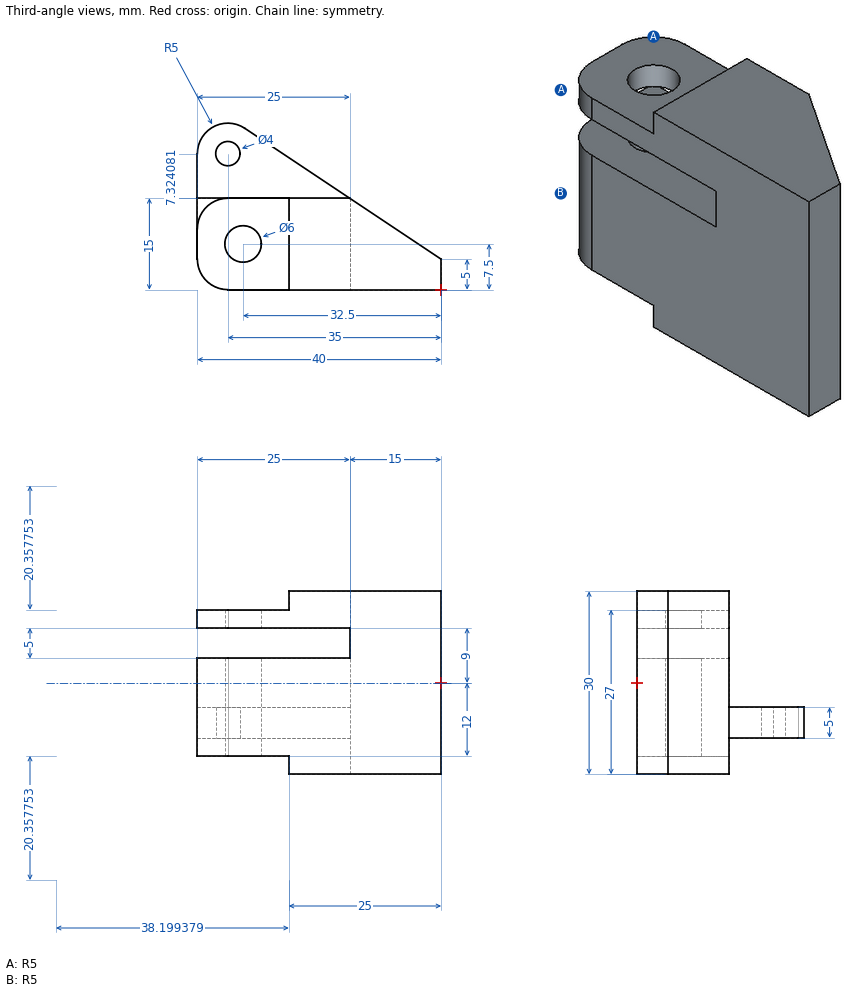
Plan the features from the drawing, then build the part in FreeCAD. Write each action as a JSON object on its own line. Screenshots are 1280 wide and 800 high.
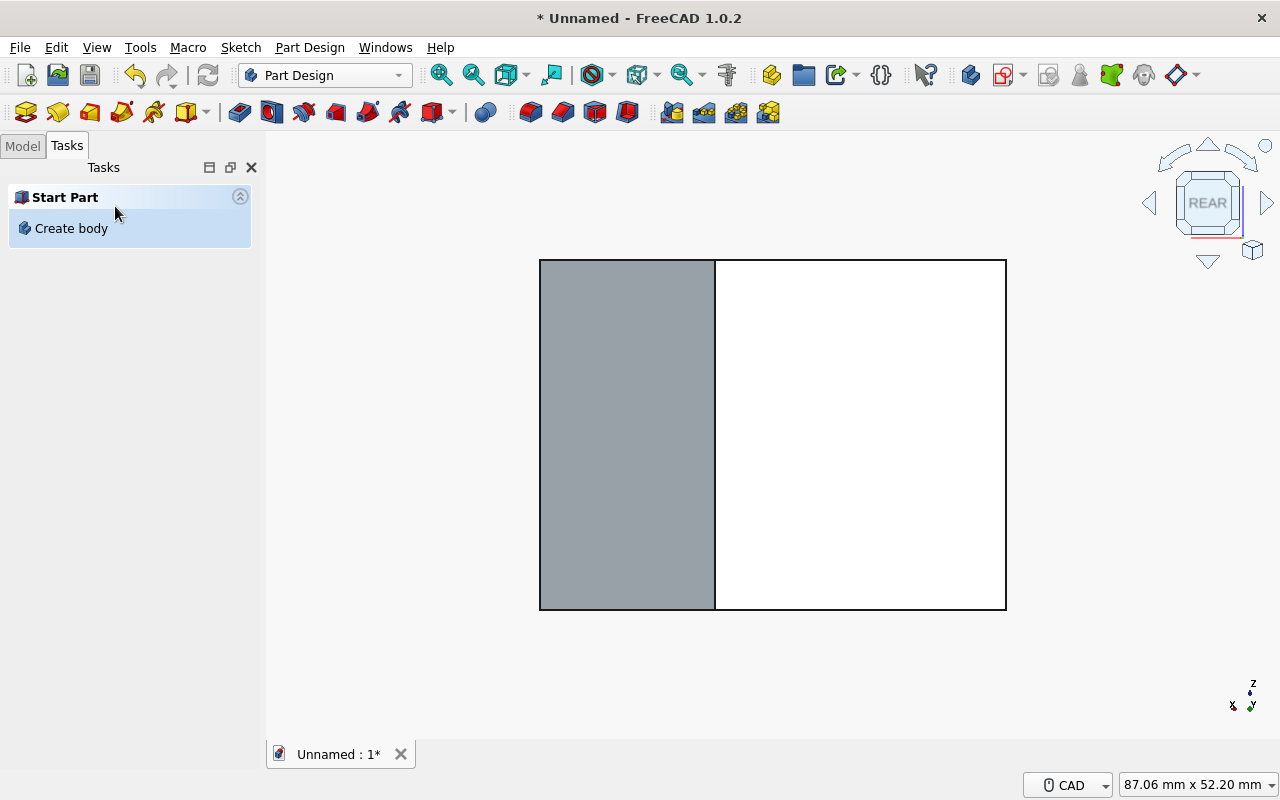
{"action": "left_click", "coordinate": [860, 434]}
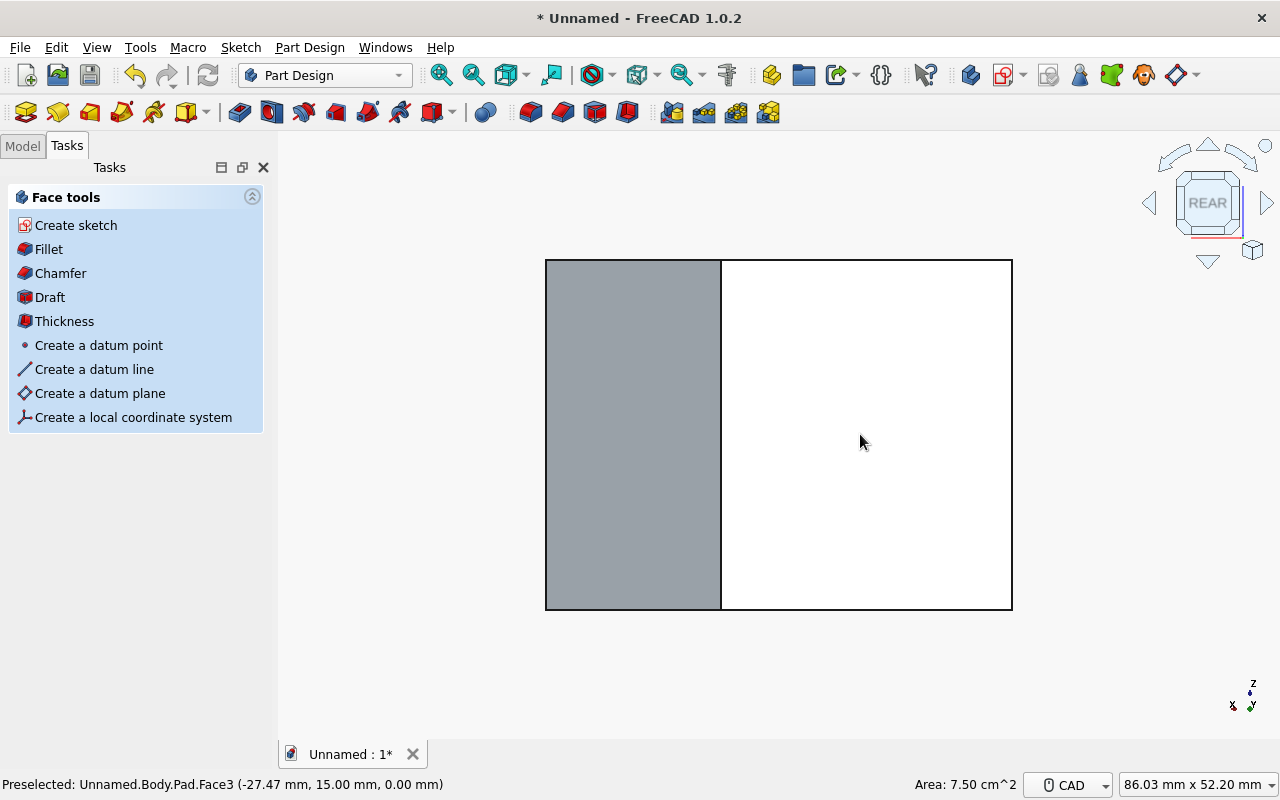
{"action": "left_click", "coordinate": [1004, 76]}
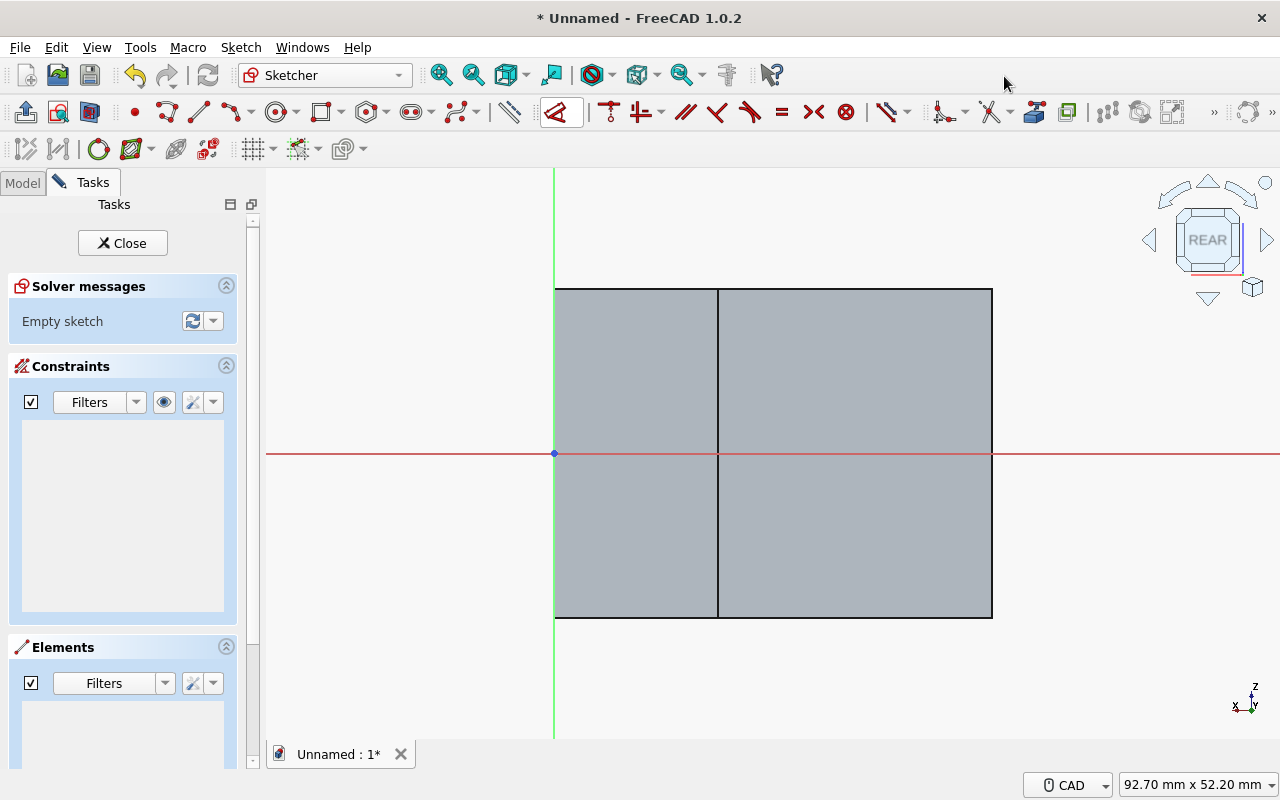
{"action": "scroll", "coordinate": [467, 454], "scroll_direction": "down", "scroll_amount": 3}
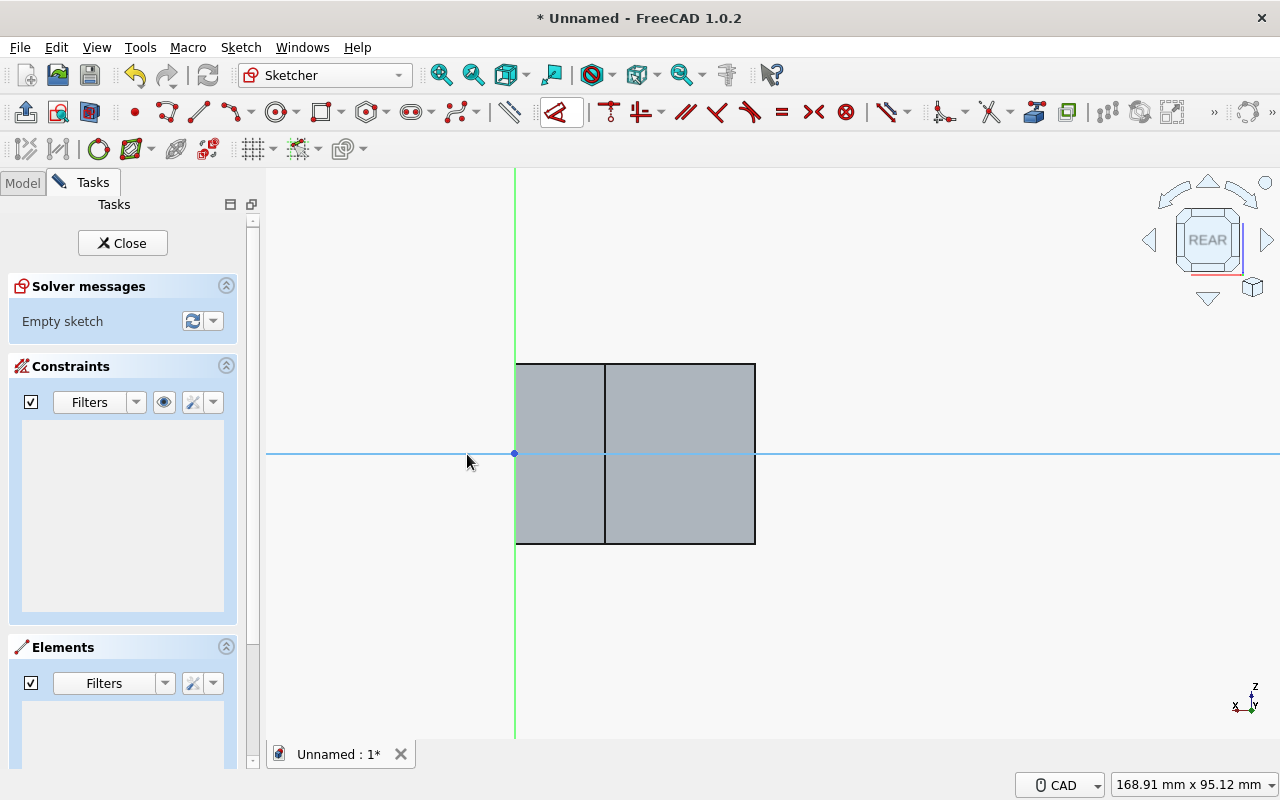
{"action": "key", "text": "g r"}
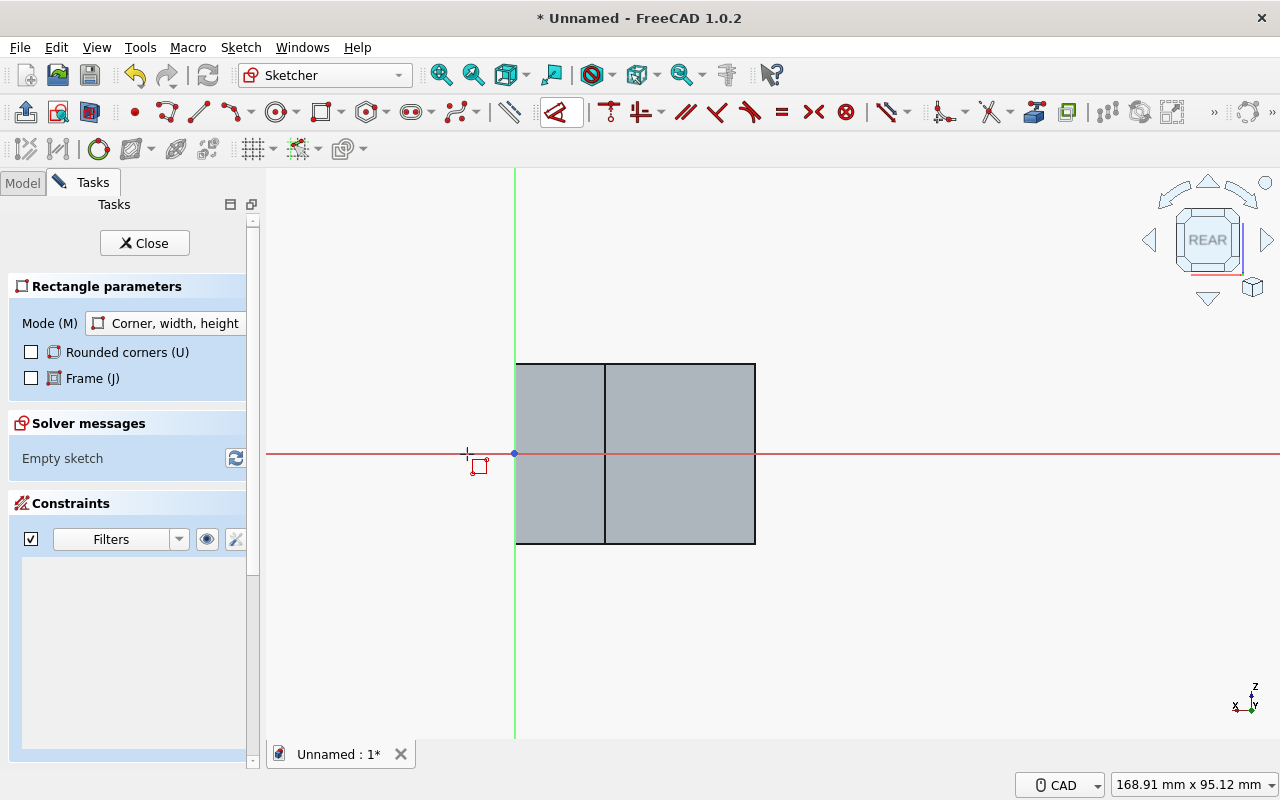
{"action": "left_click", "coordinate": [665, 526]}
{"action": "mouse_move", "coordinate": [894, 648]}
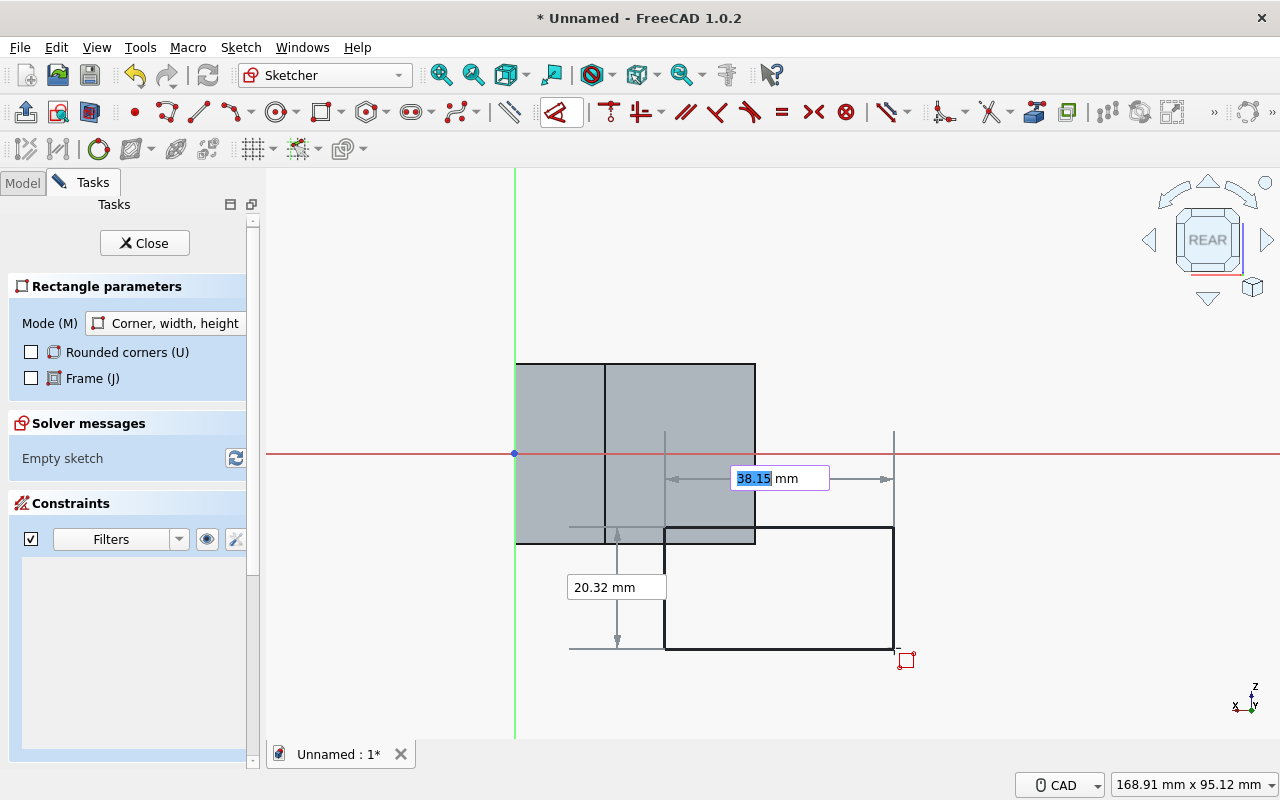
{"action": "type", "text": "38.199379"}
{"action": "key", "text": "Tab"}
{"action": "type", "text": "20.357753"}
{"action": "key", "text": "Return"}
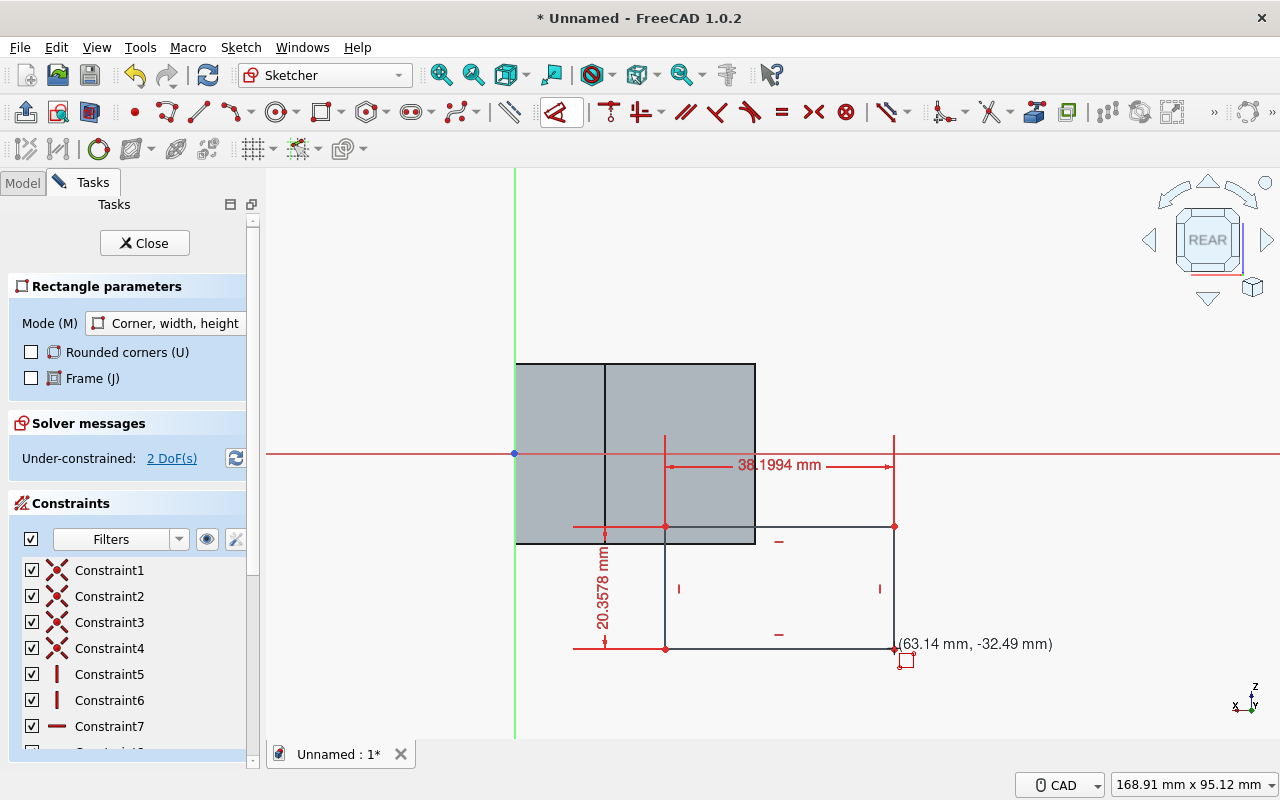
{"action": "left_click", "coordinate": [665, 260]}
{"action": "mouse_move", "coordinate": [894, 382]}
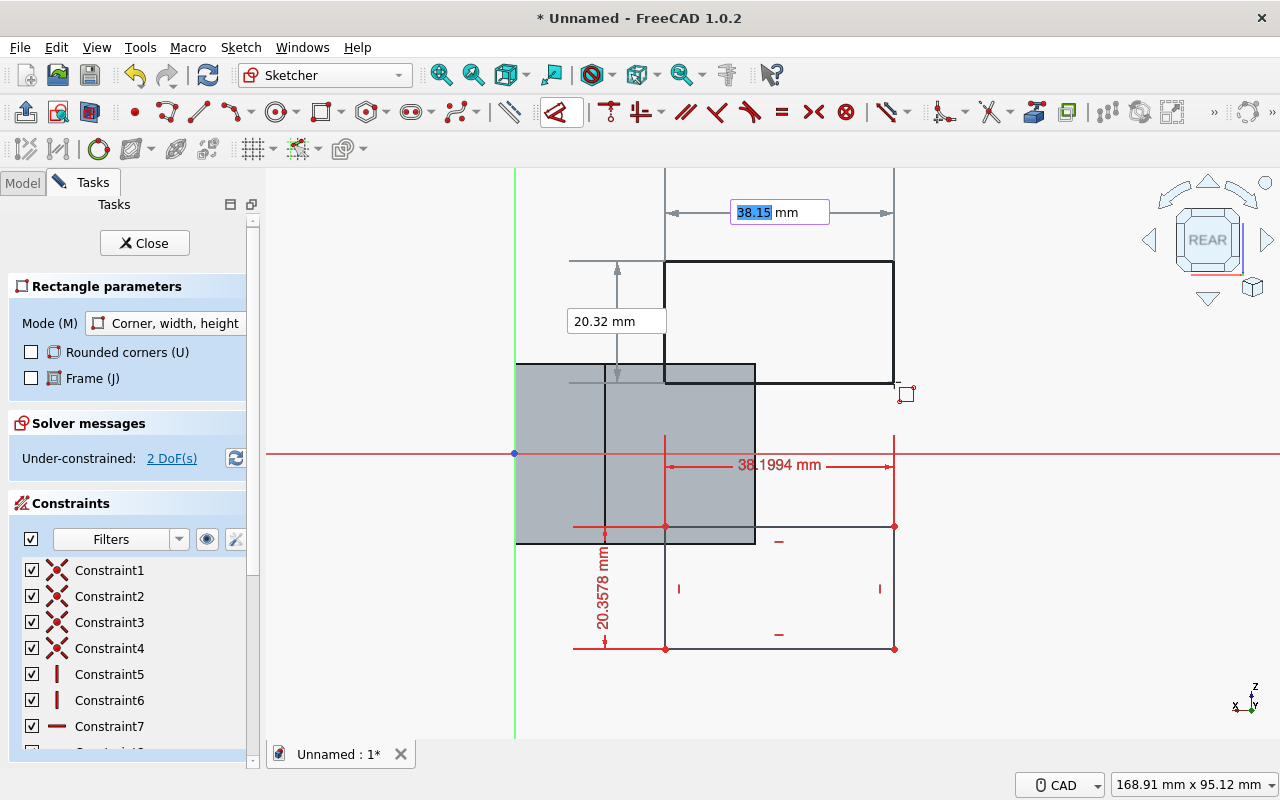
{"action": "type", "text": "38.199379"}
{"action": "key", "text": "Tab"}
{"action": "type", "text": "20.357753"}
{"action": "key", "text": "Return"}
{"action": "key", "text": "Escape"}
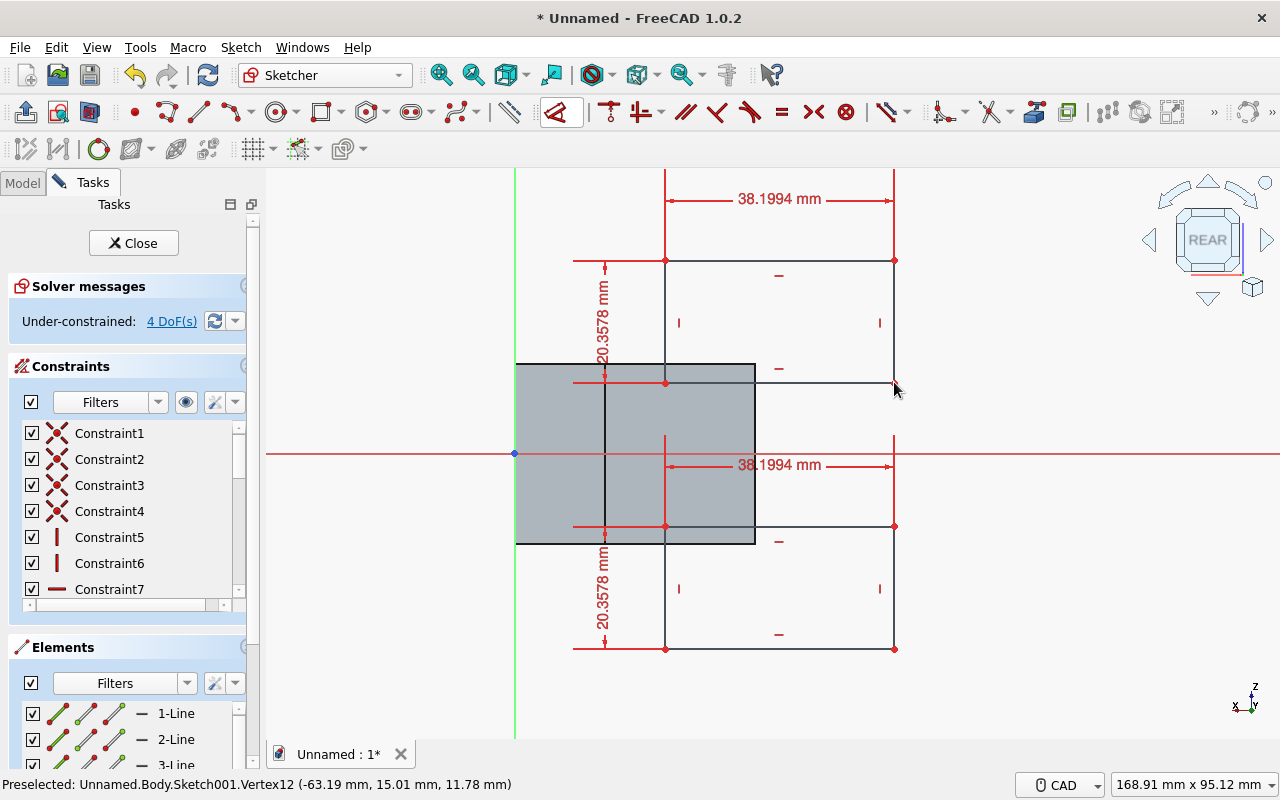
{"action": "left_click", "coordinate": [665, 649]}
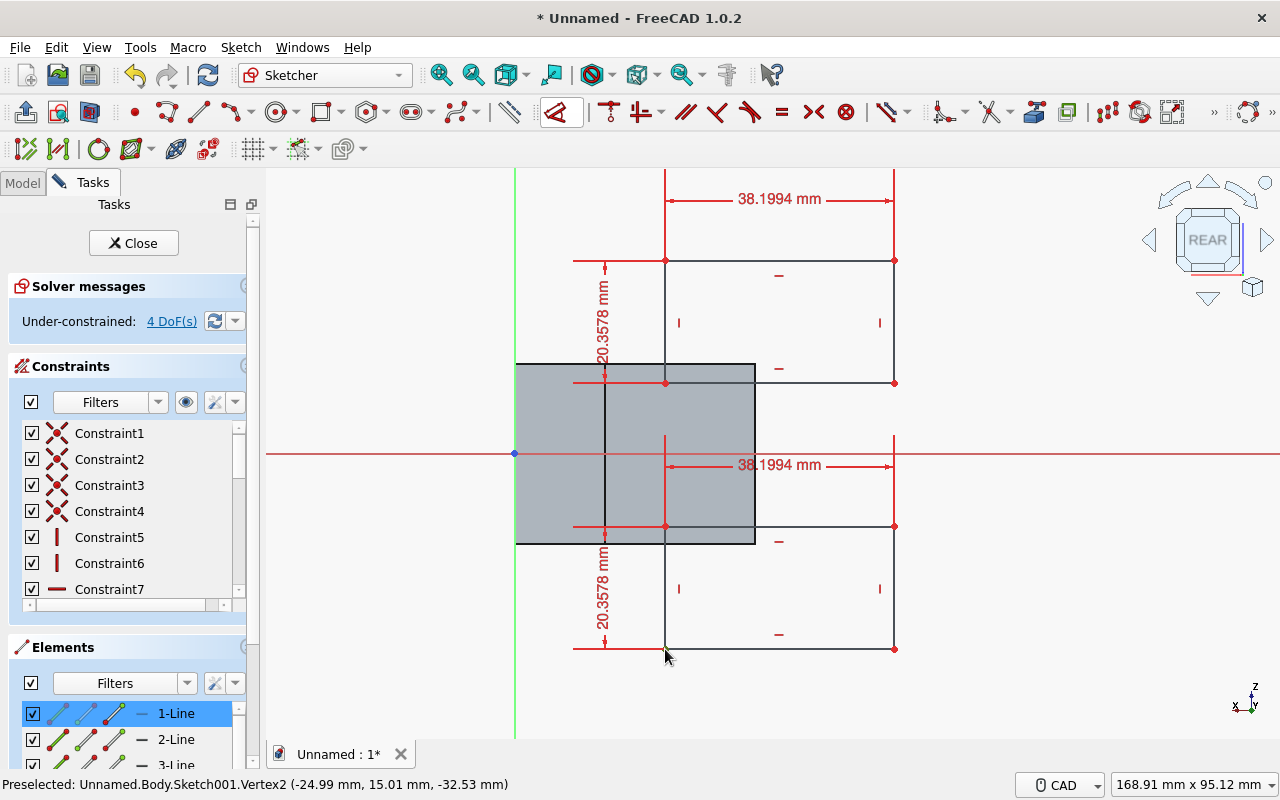
{"action": "left_click", "coordinate": [665, 261]}